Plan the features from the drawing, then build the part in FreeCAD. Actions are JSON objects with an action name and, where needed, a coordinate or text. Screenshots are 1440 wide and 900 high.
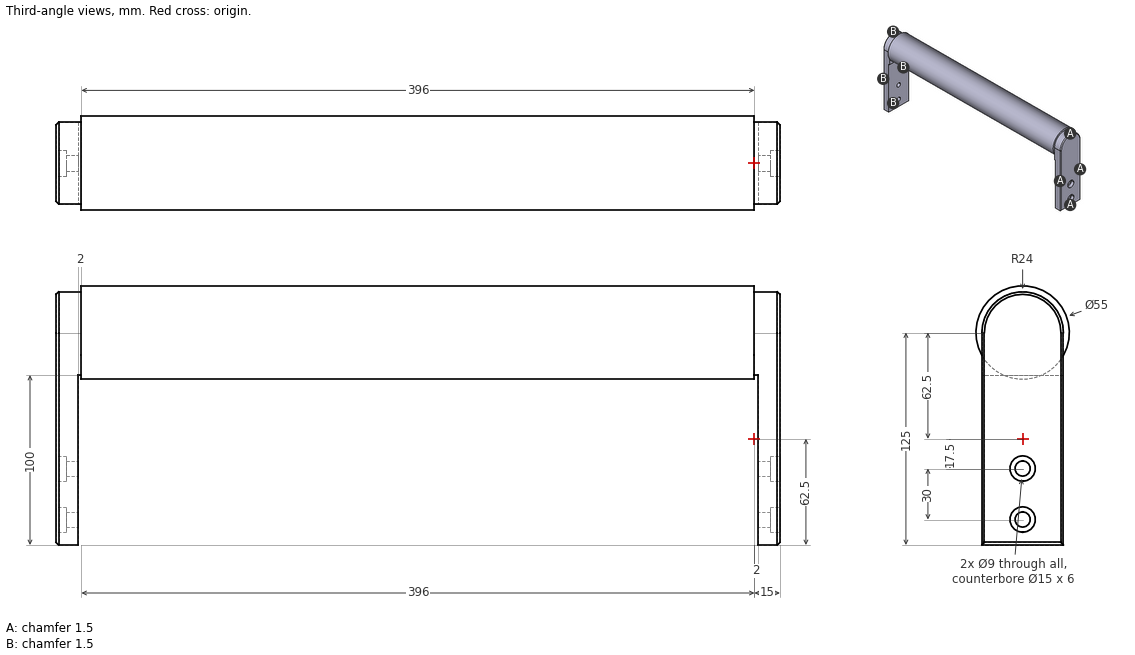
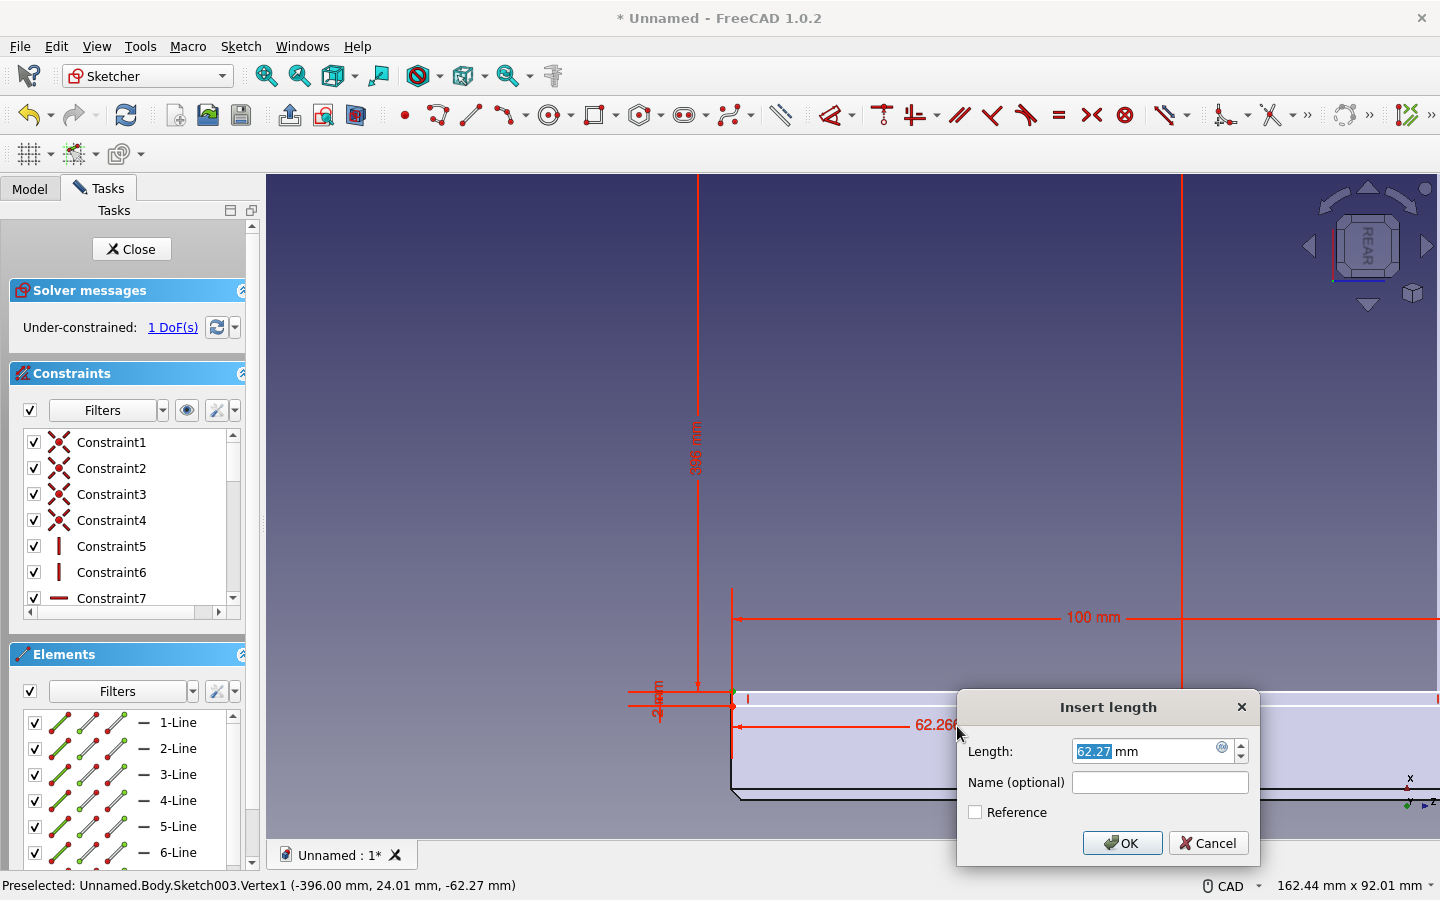
{"action": "type", "text": "62.5"}
{"action": "key", "text": "Return"}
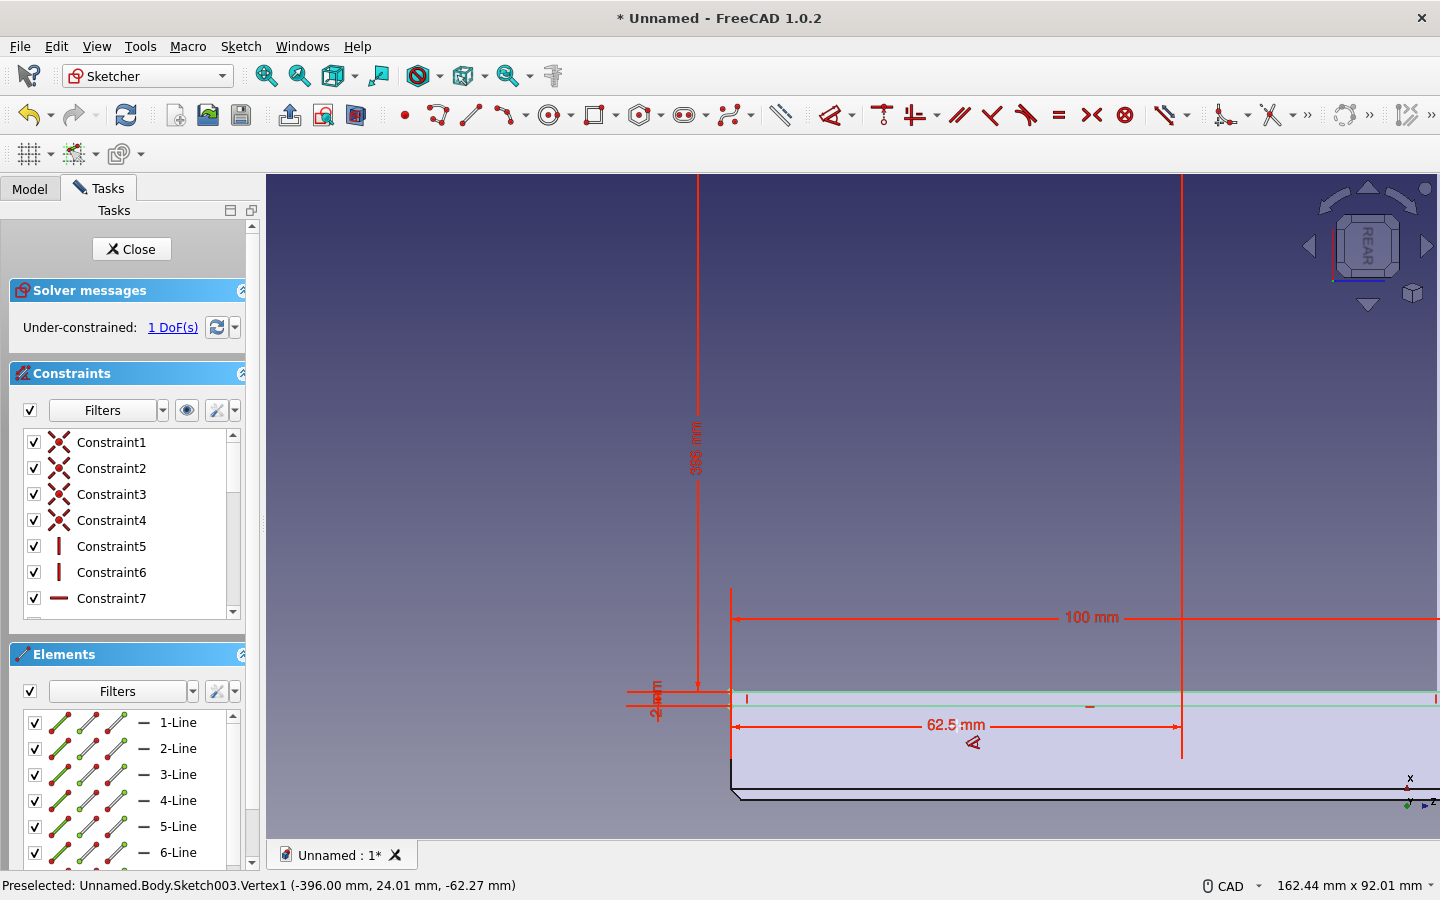
{"action": "scroll", "coordinate": [736, 701], "scroll_direction": "down", "scroll_amount": 10}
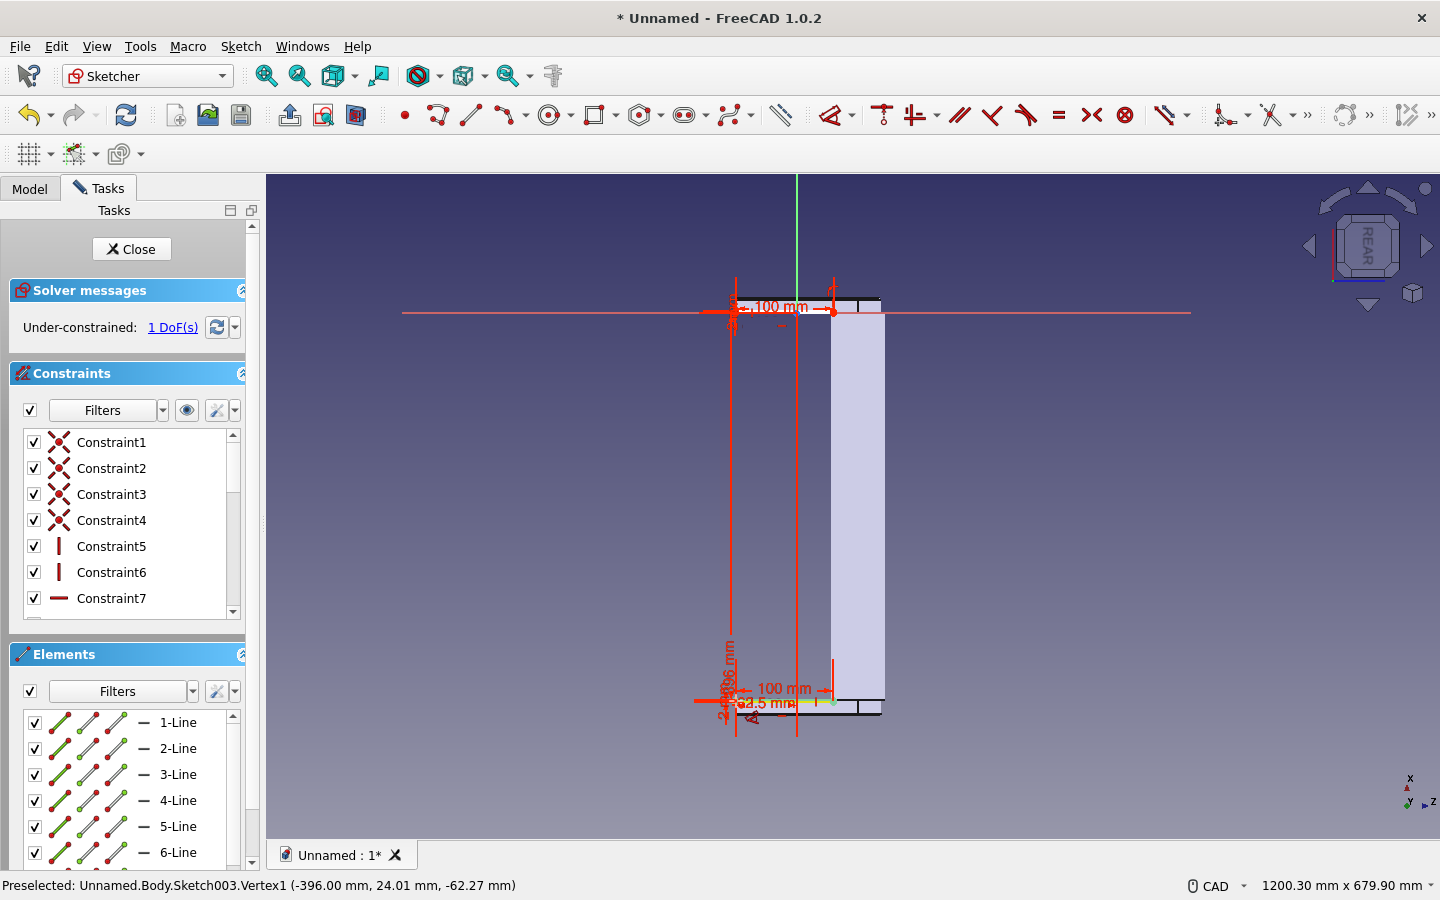
{"action": "scroll", "coordinate": [736, 311], "scroll_direction": "up", "scroll_amount": 10}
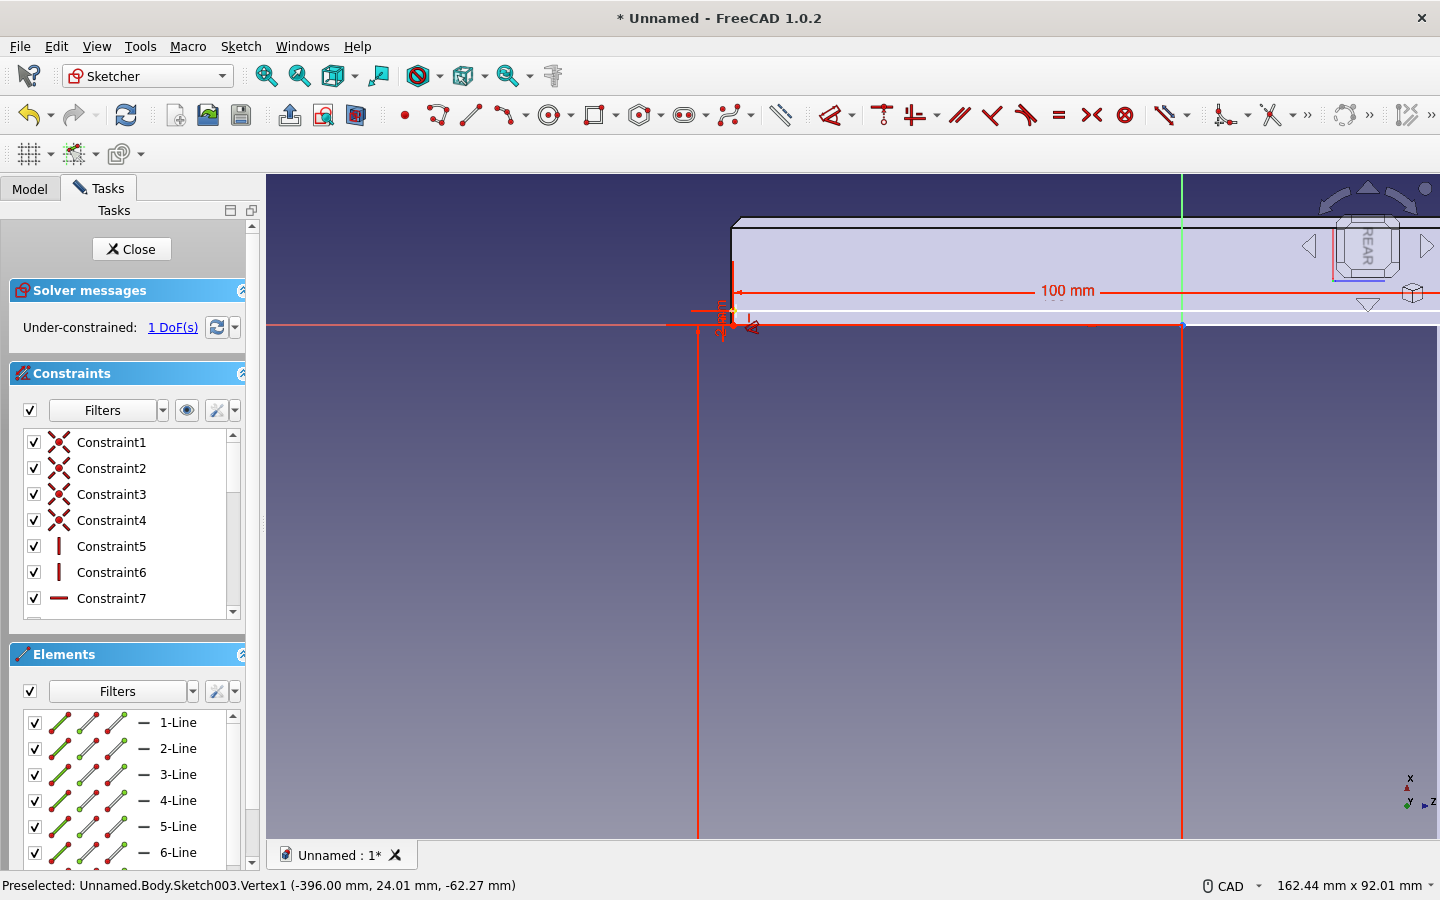
{"action": "left_click", "coordinate": [733, 311]}
{"action": "left_click", "coordinate": [958, 277]}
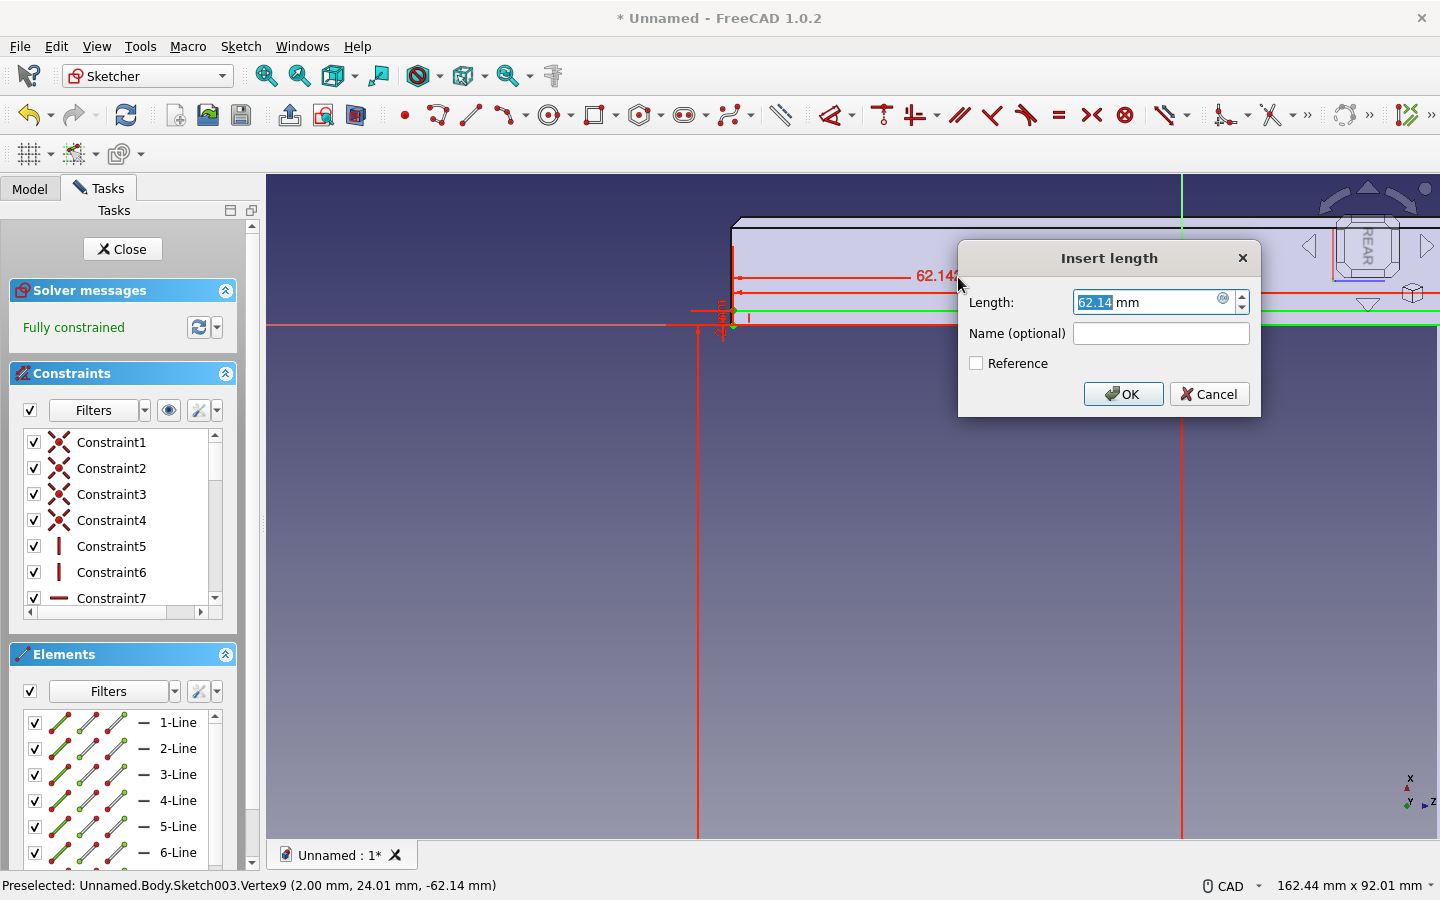
{"action": "type", "text": "62.5"}
{"action": "key", "text": "Return"}
{"action": "key", "text": "Escape"}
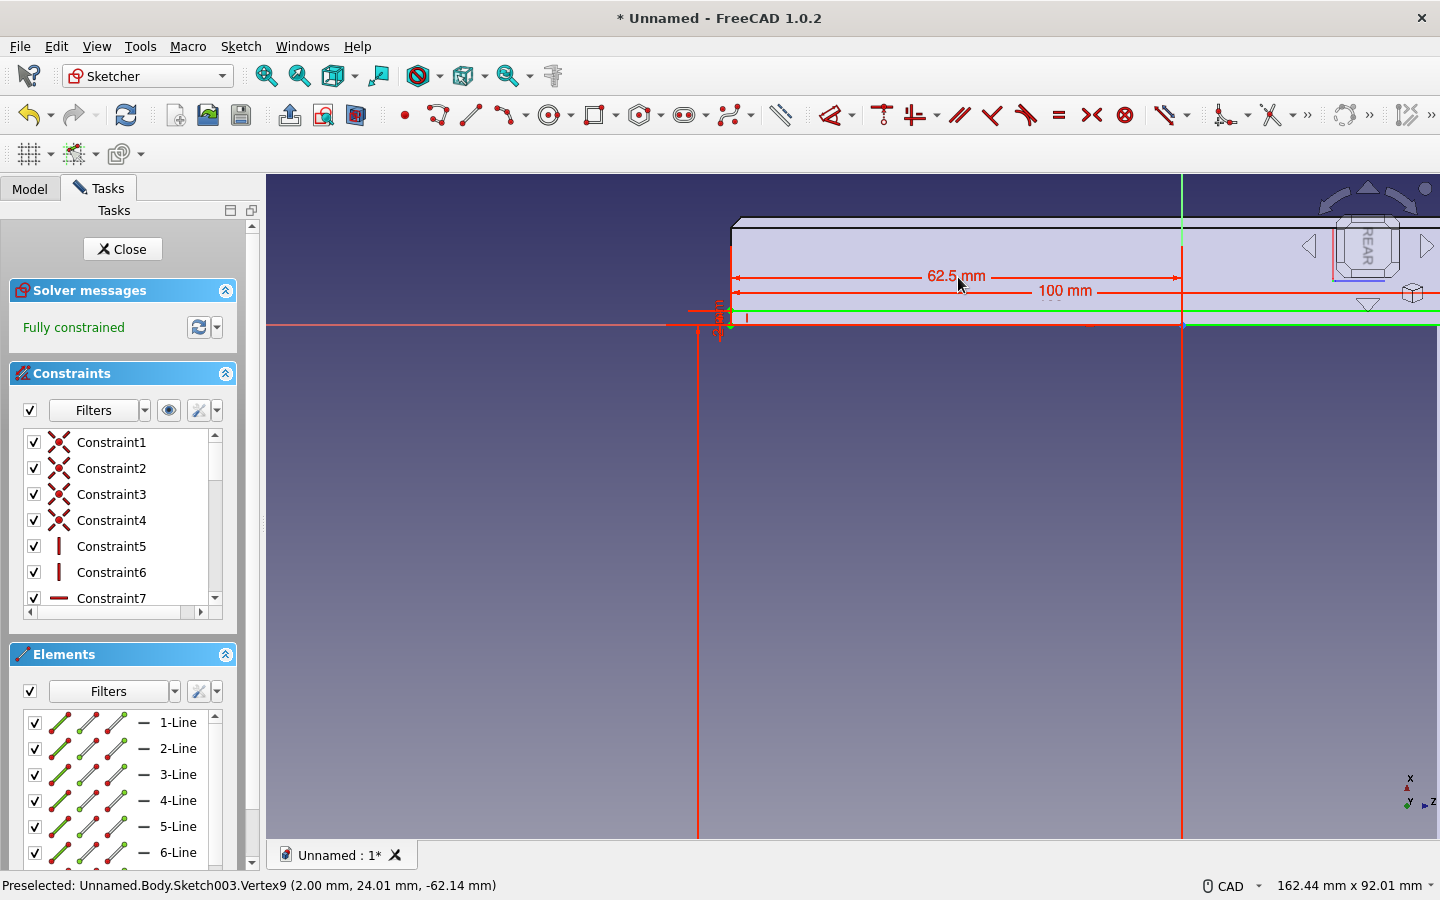
{"action": "left_click", "coordinate": [123, 249]}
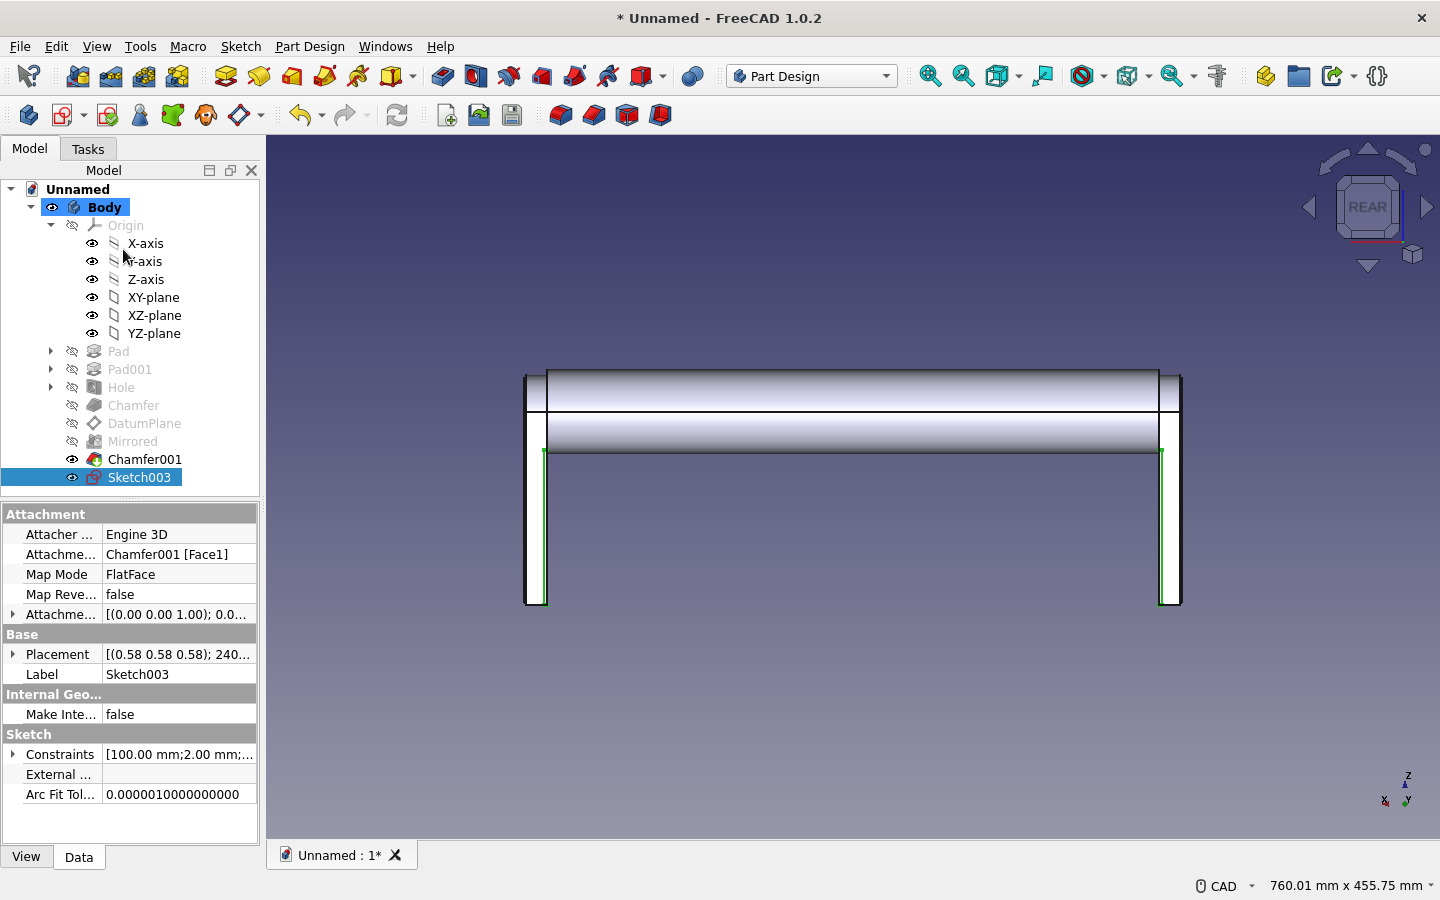
{"action": "left_click", "coordinate": [443, 76]}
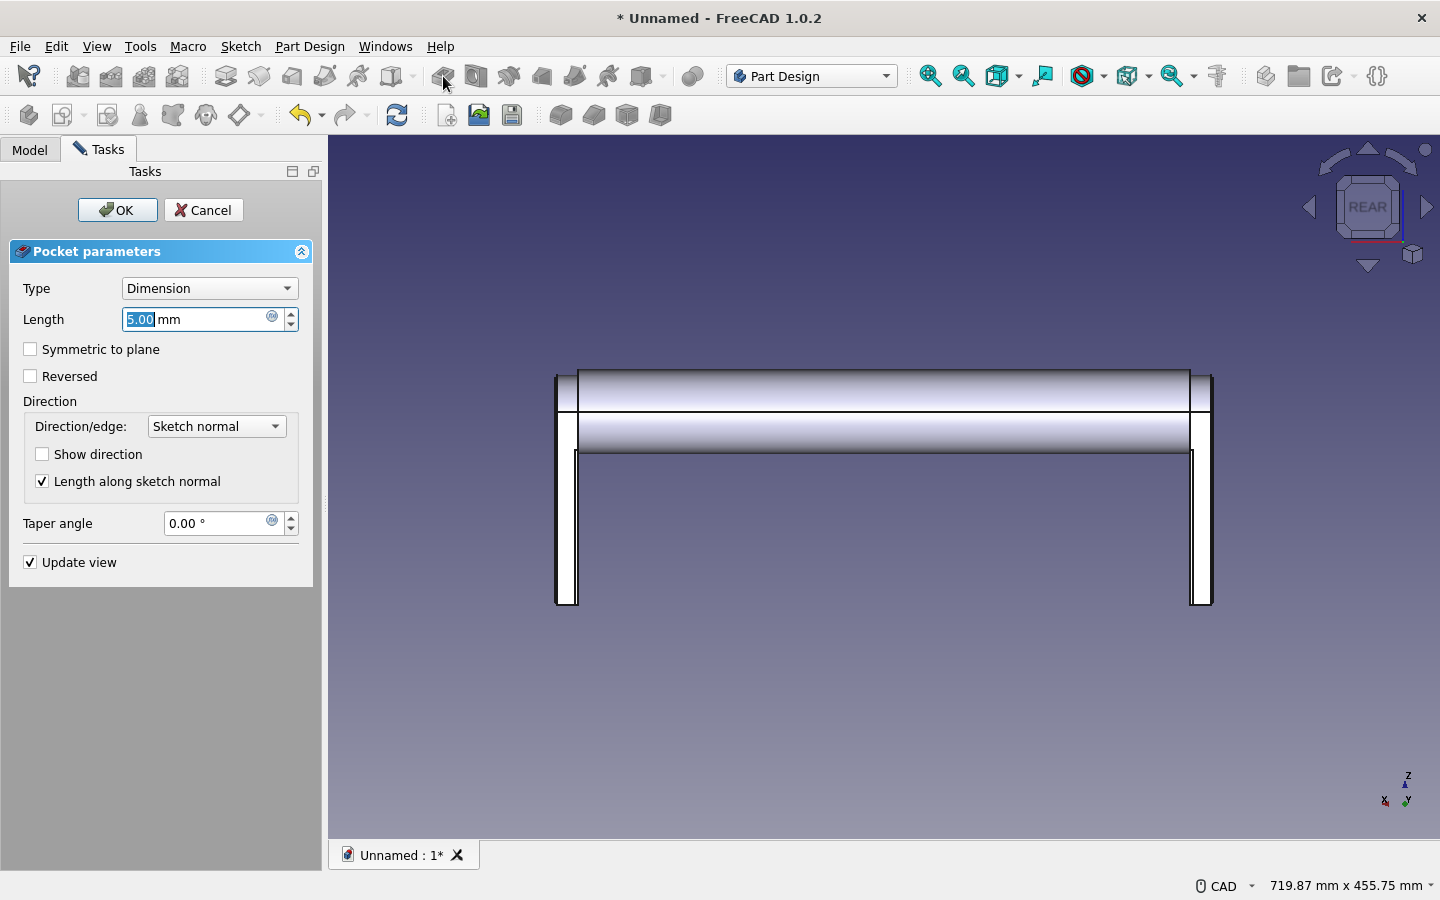
{"action": "left_click", "coordinate": [210, 288]}